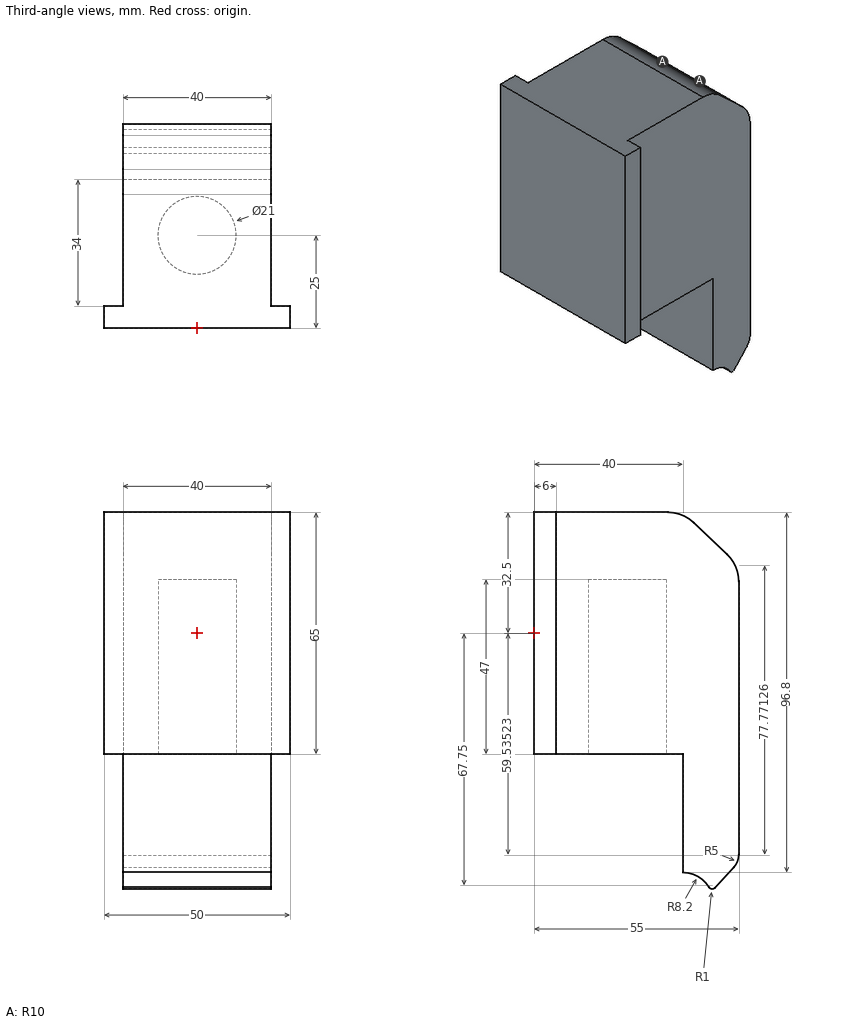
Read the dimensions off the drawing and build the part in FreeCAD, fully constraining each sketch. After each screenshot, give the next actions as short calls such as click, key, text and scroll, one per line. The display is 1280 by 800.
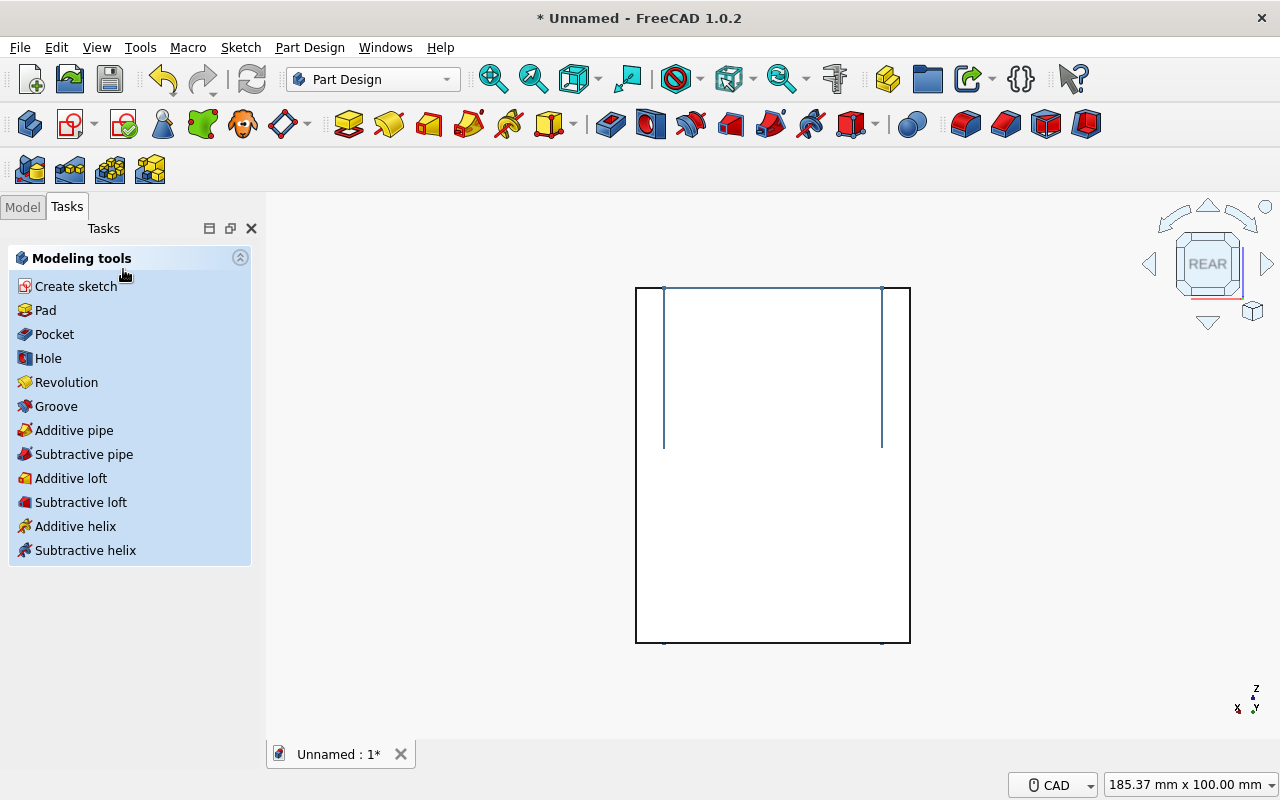
click(350, 124)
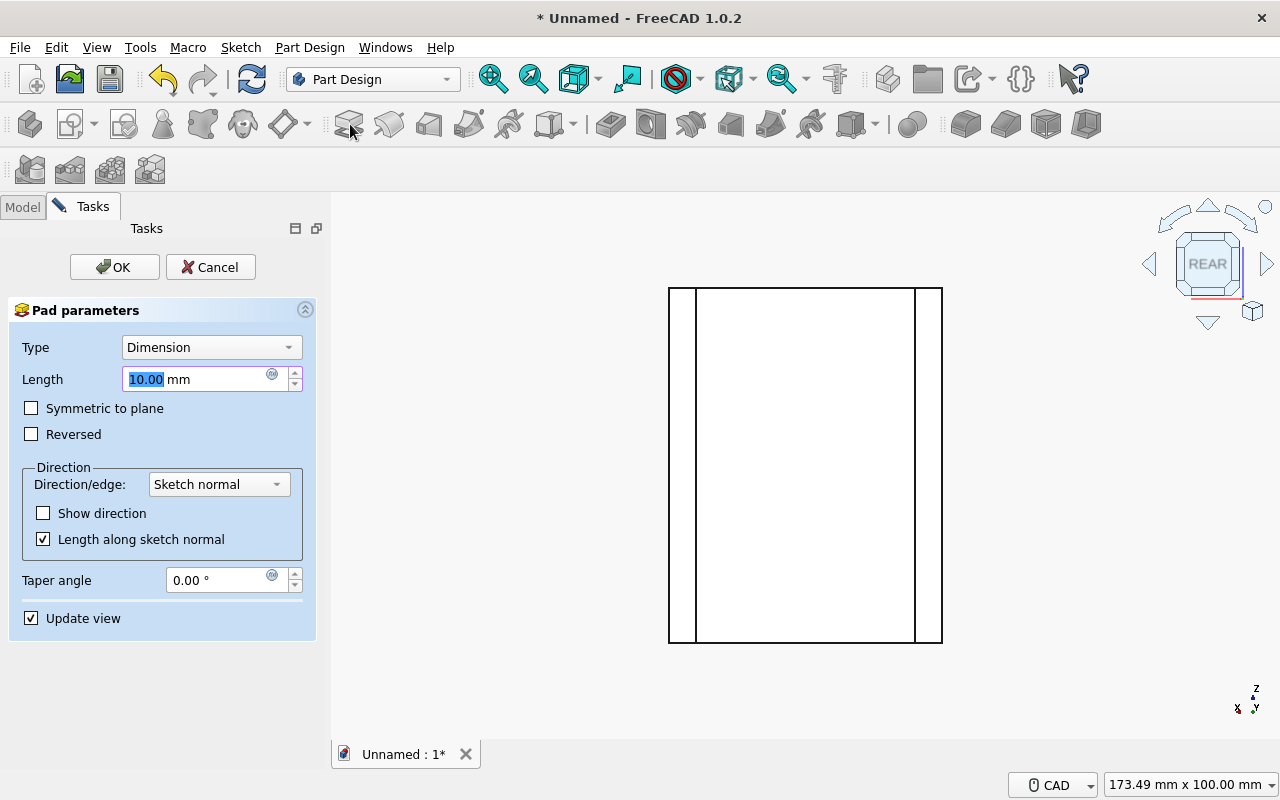
text(34)
key(Tab)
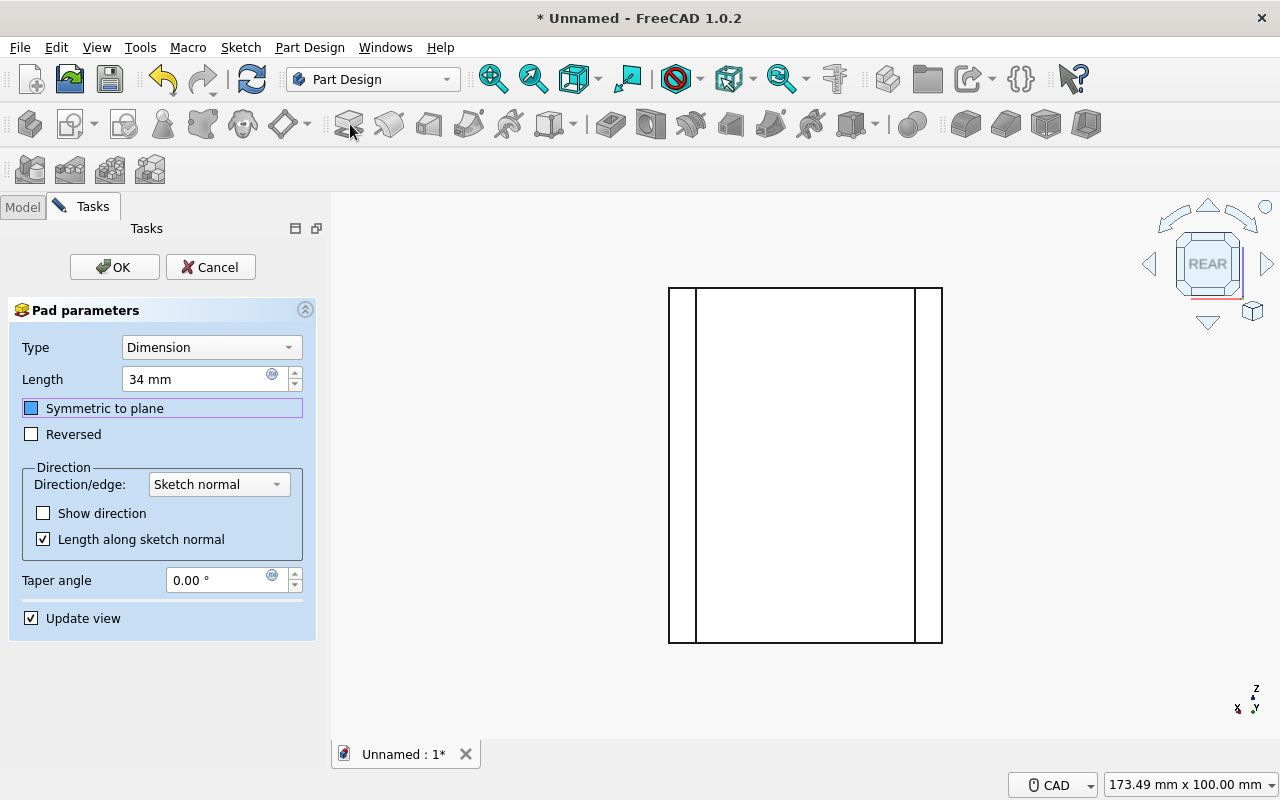
click(115, 267)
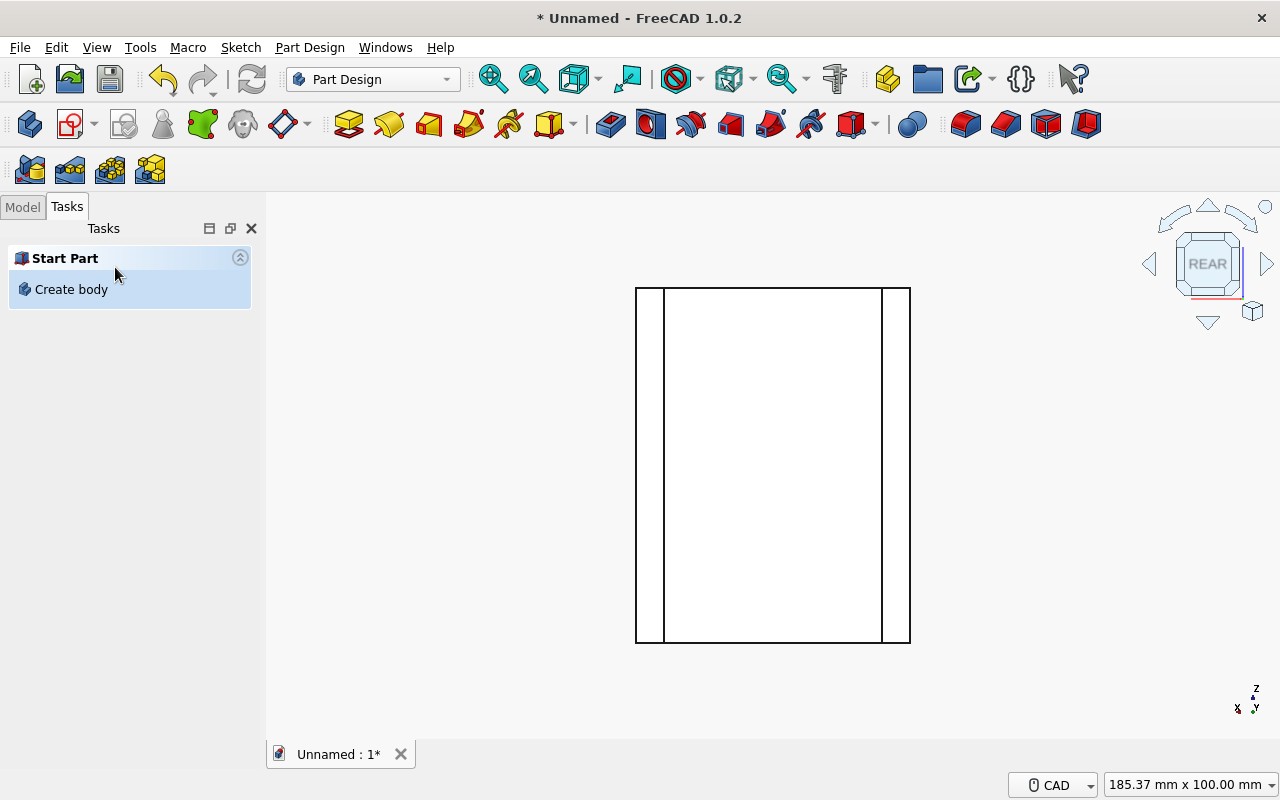
key(5)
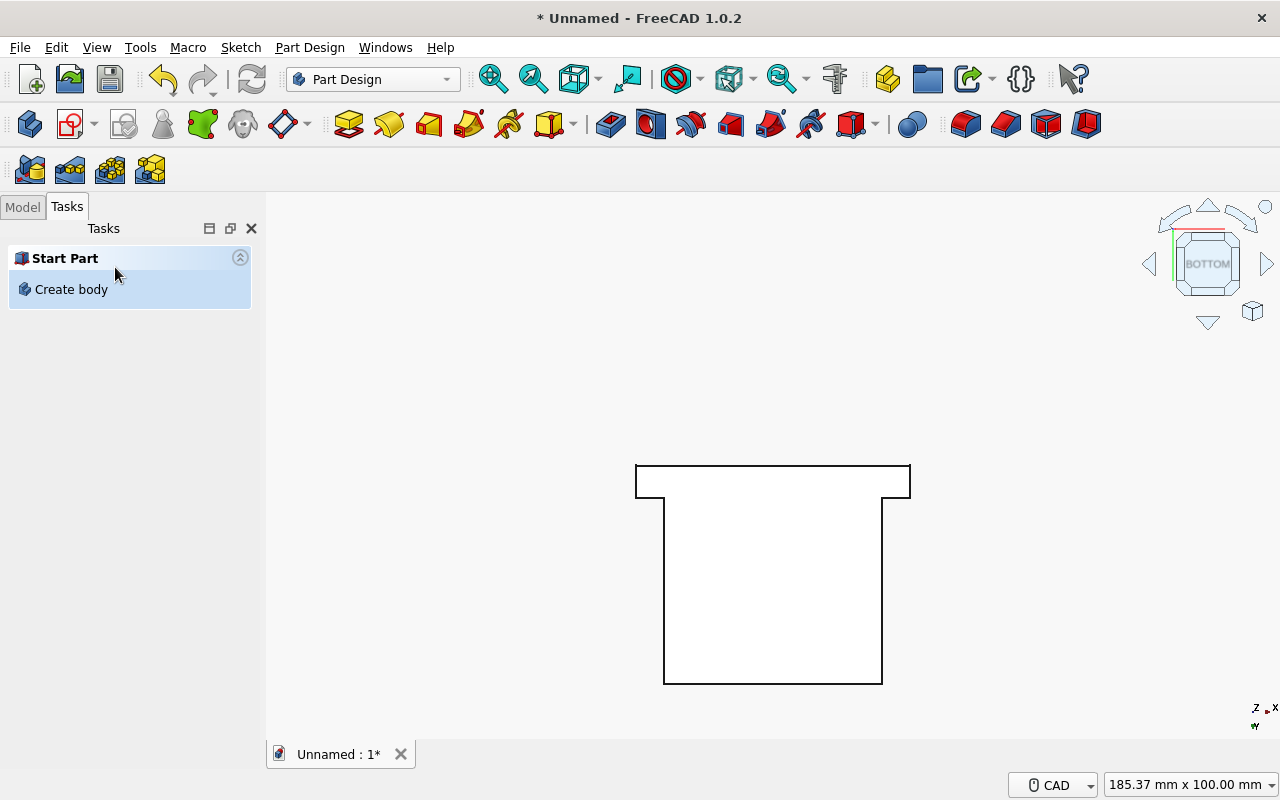
key(v)
key(f)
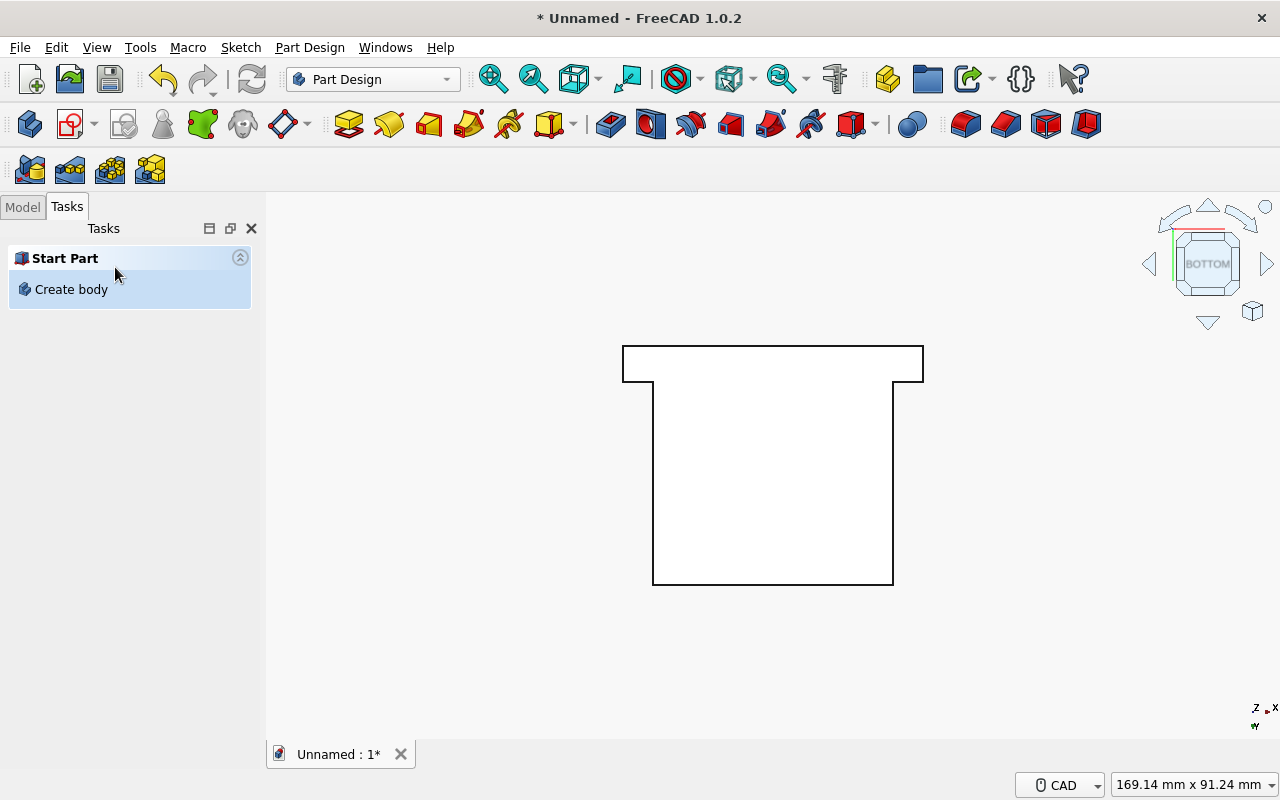
click(773, 464)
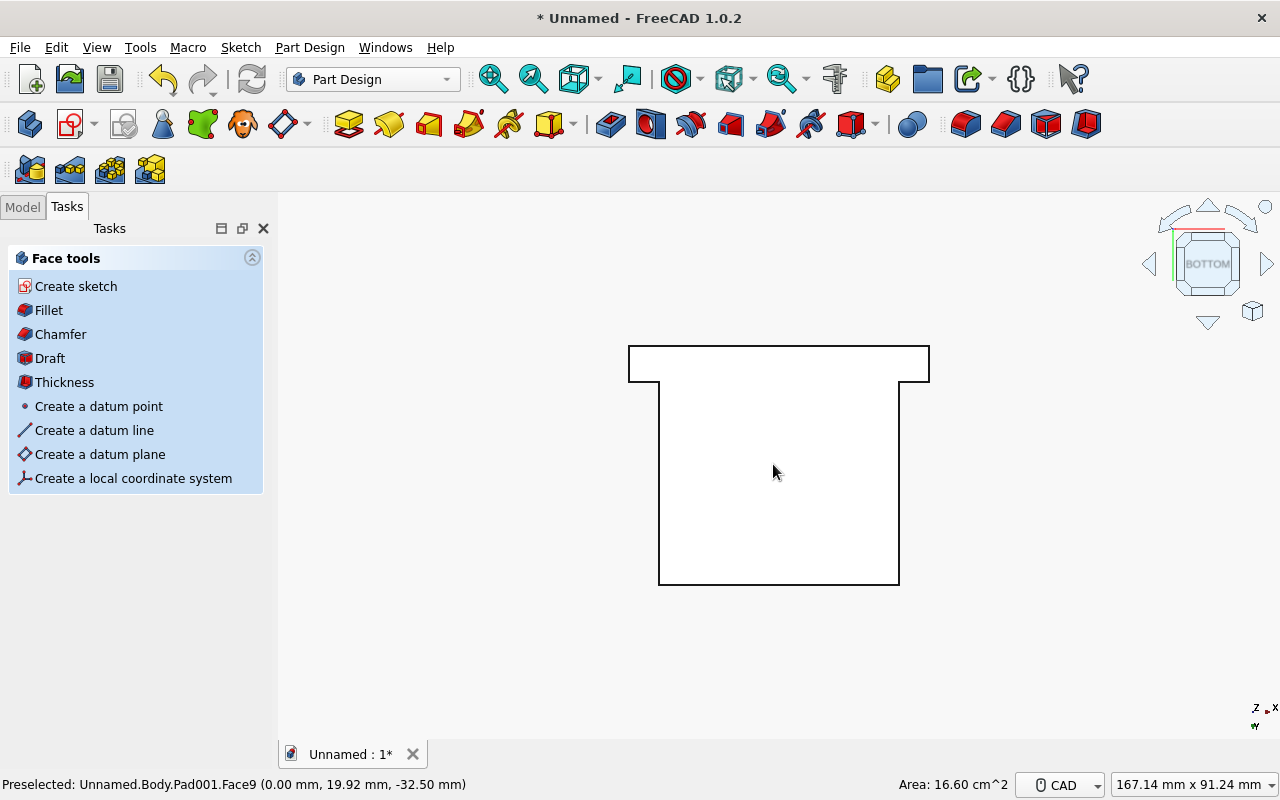
click(70, 124)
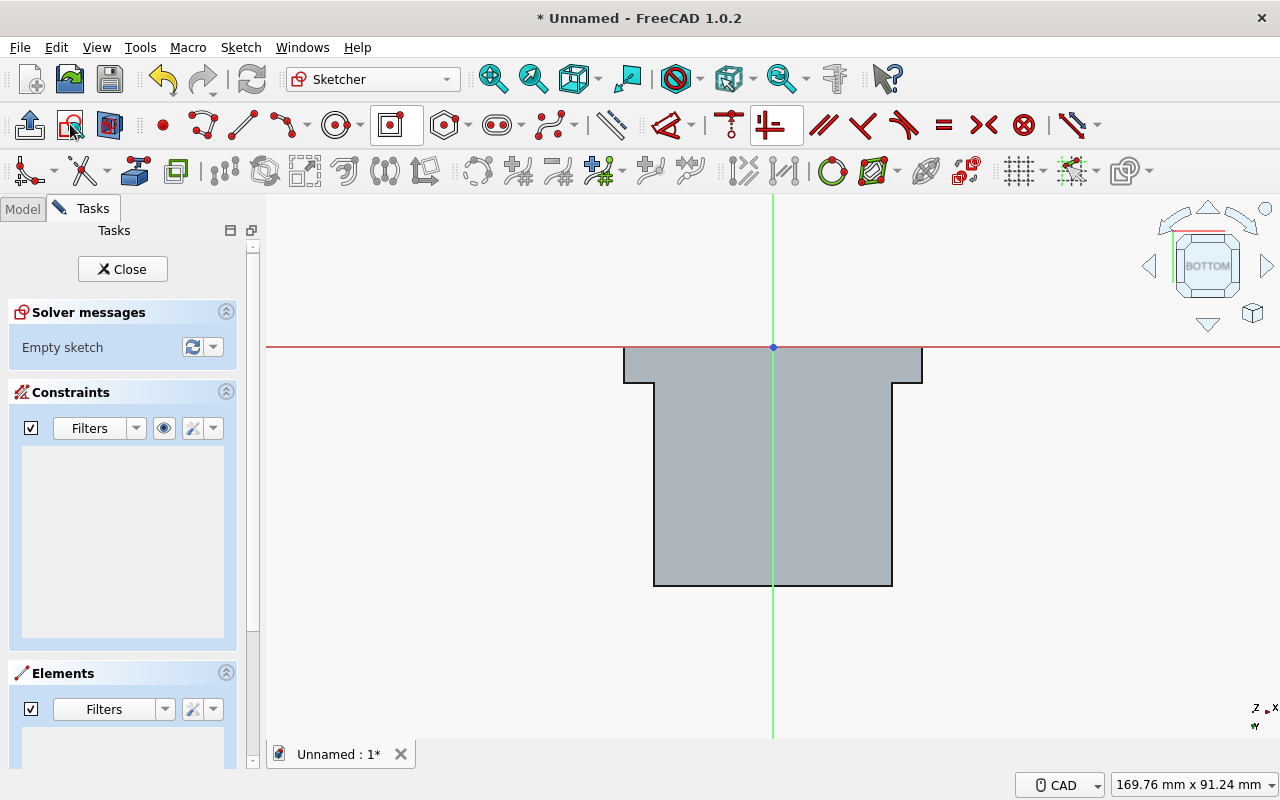
scroll(912, 426, up, 2)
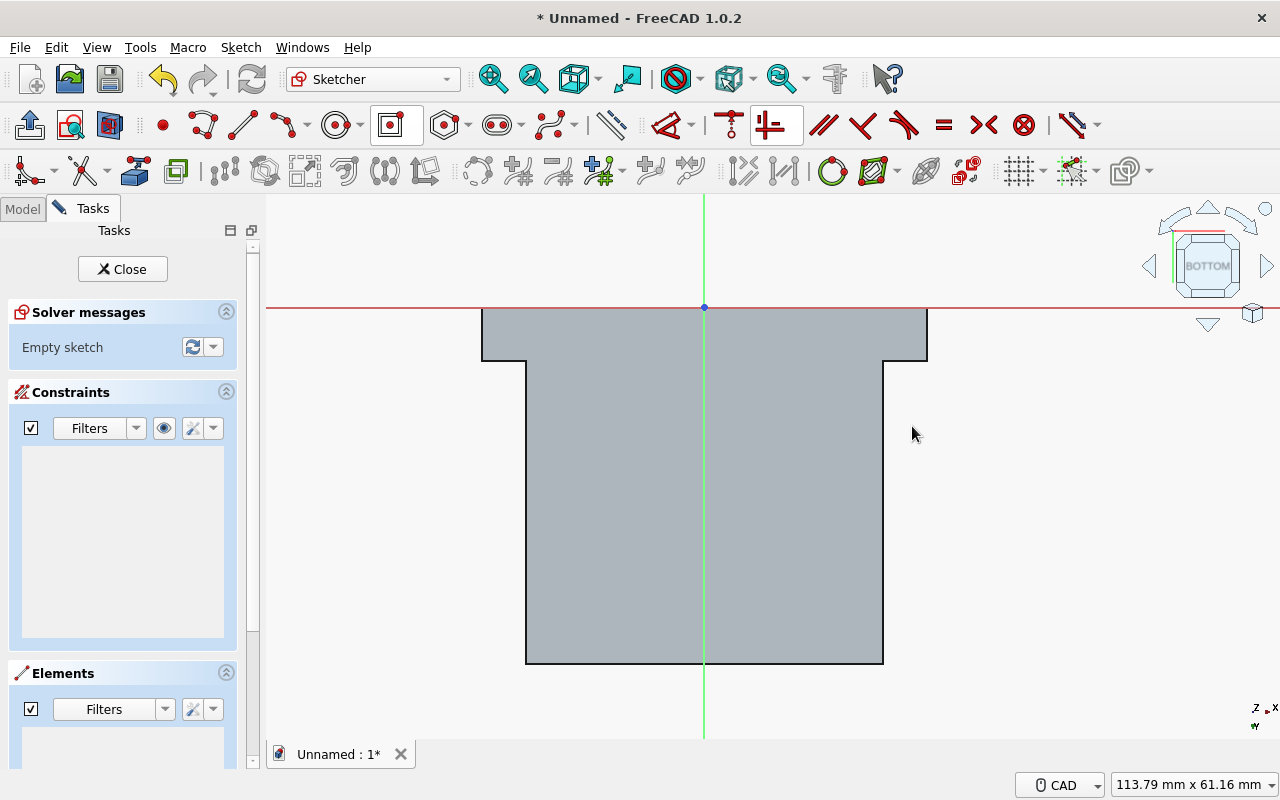
click(336, 126)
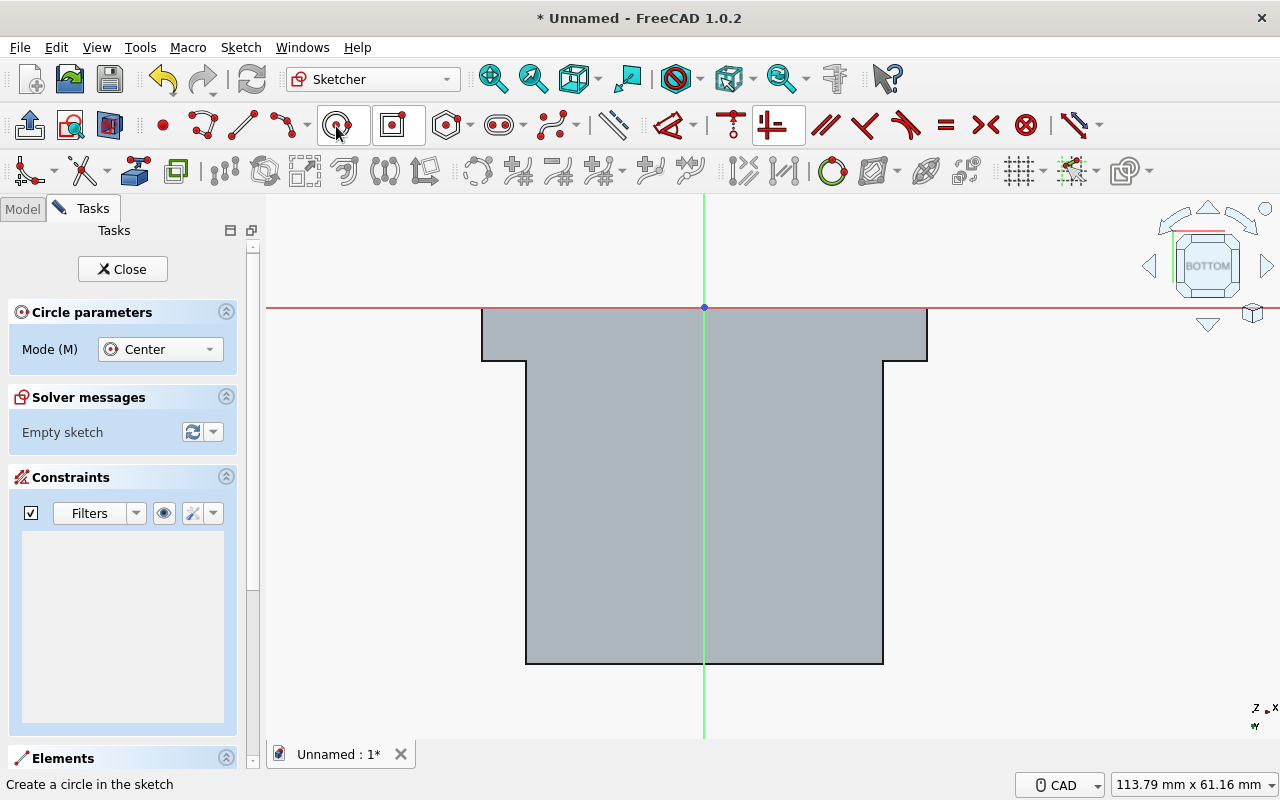
click(704, 531)
move(770, 465)